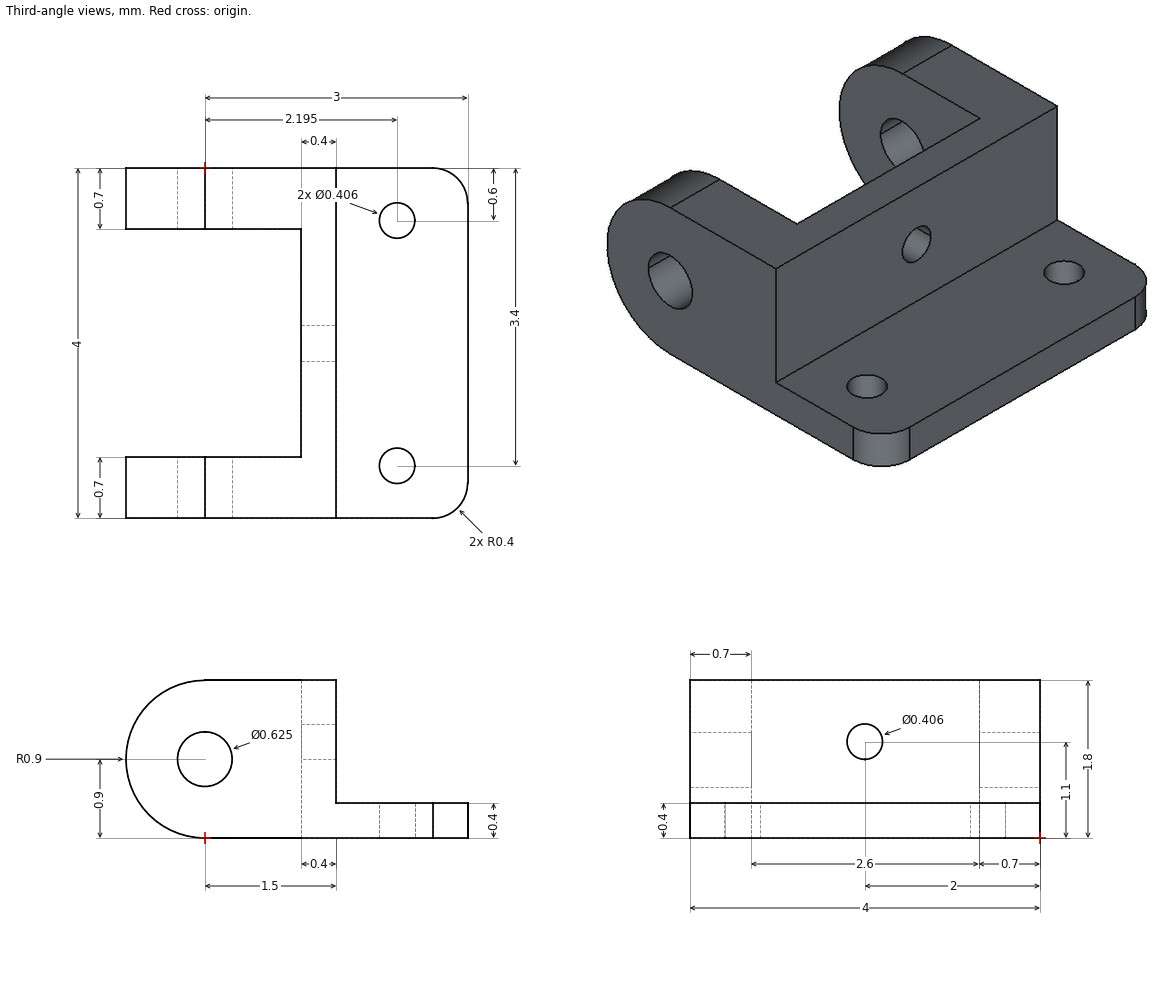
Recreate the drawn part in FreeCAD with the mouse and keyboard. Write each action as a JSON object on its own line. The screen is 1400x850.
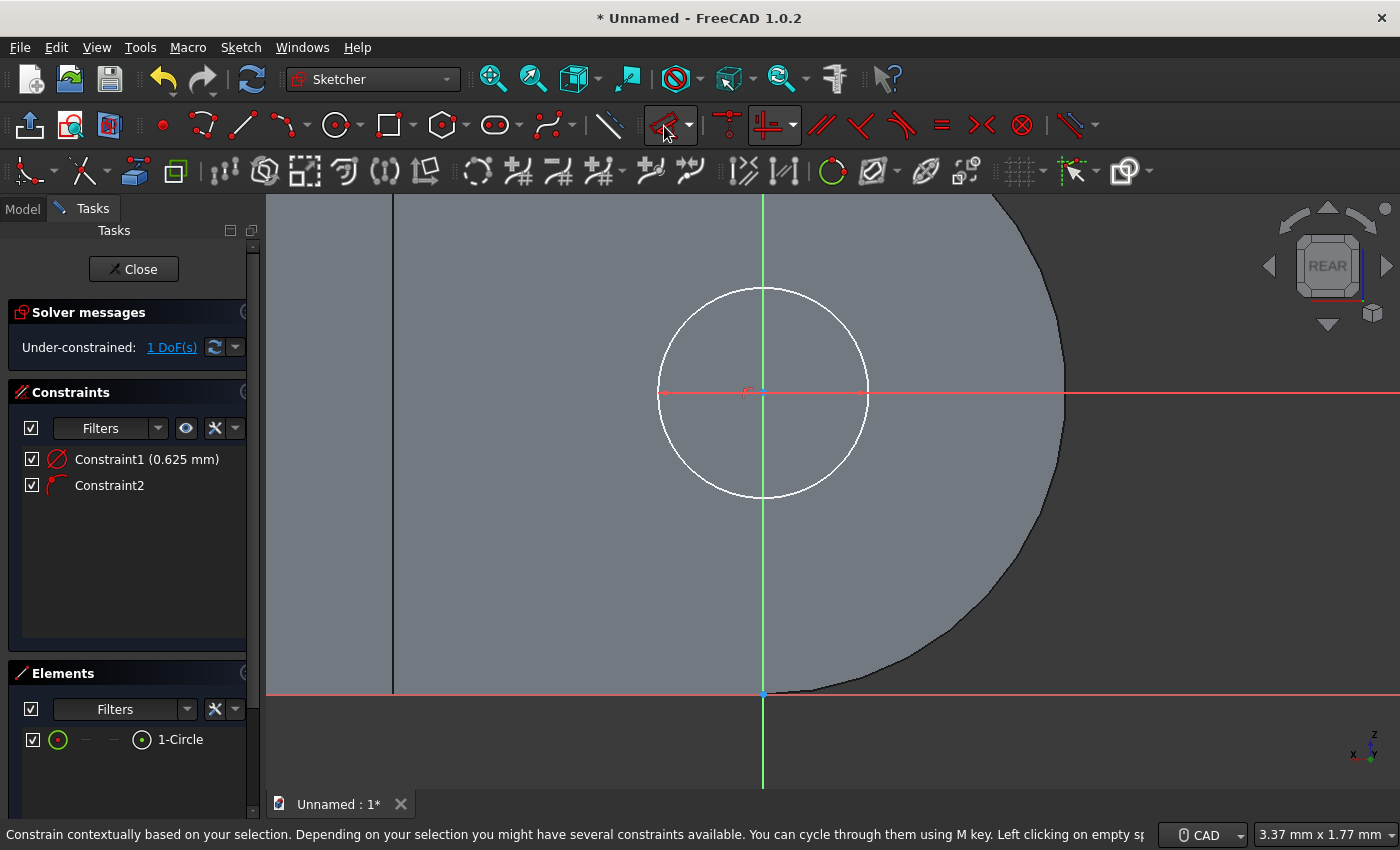
{"action": "left_click", "coordinate": [763, 393]}
{"action": "left_click", "coordinate": [797, 544]}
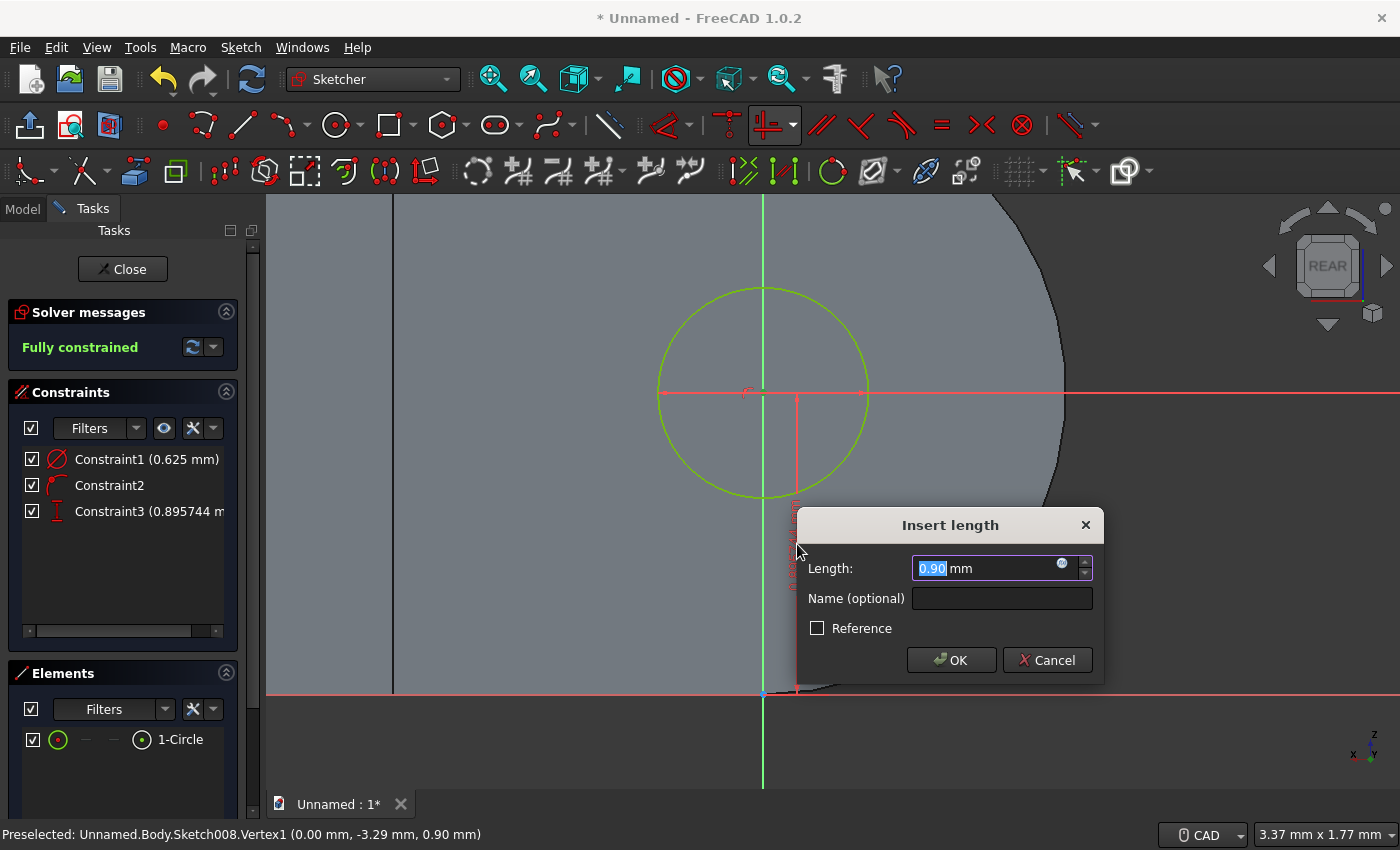
{"action": "type", "text": "0.9"}
{"action": "key", "text": "Return"}
{"action": "key", "text": "Escape"}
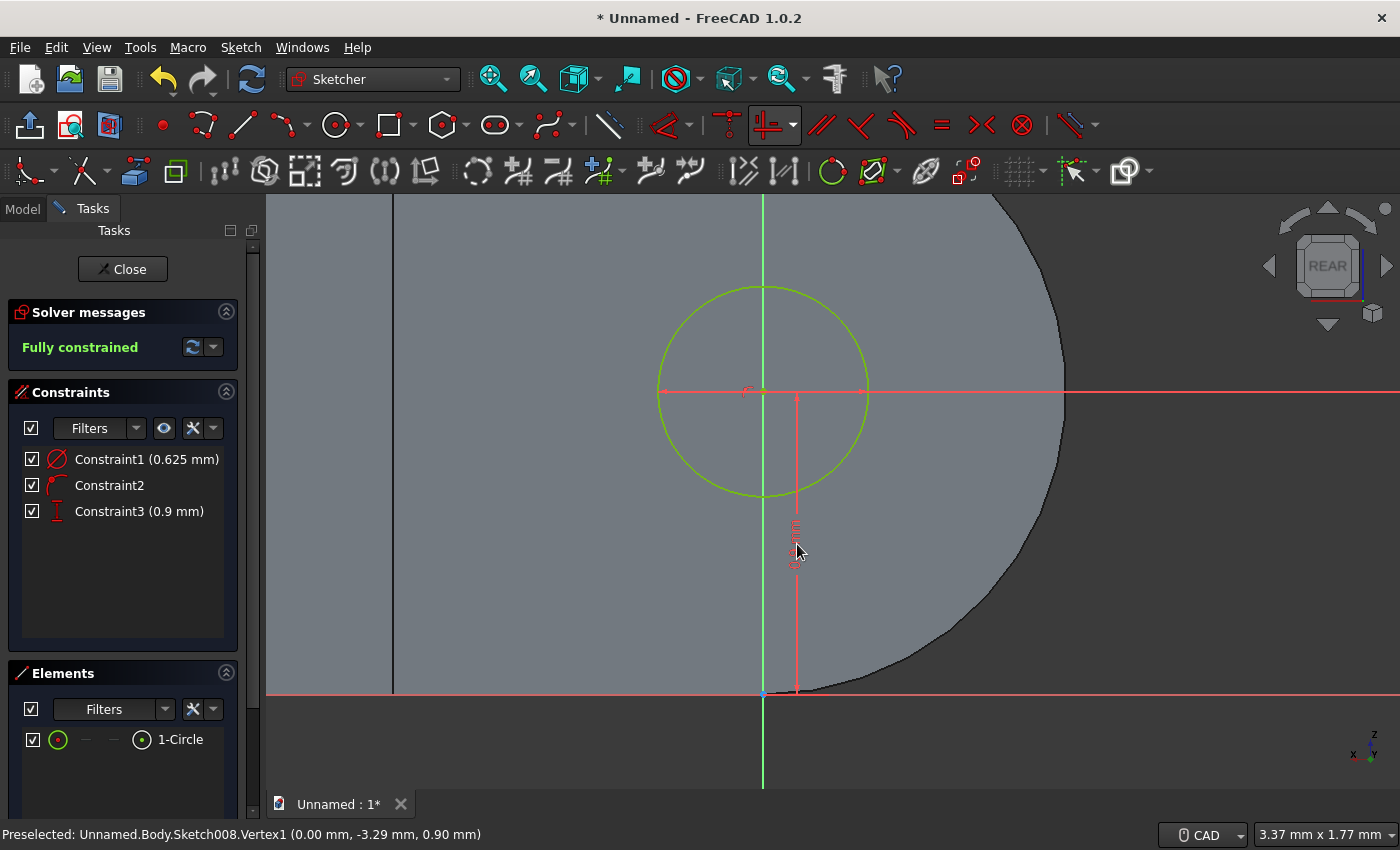
{"action": "left_click", "coordinate": [123, 269]}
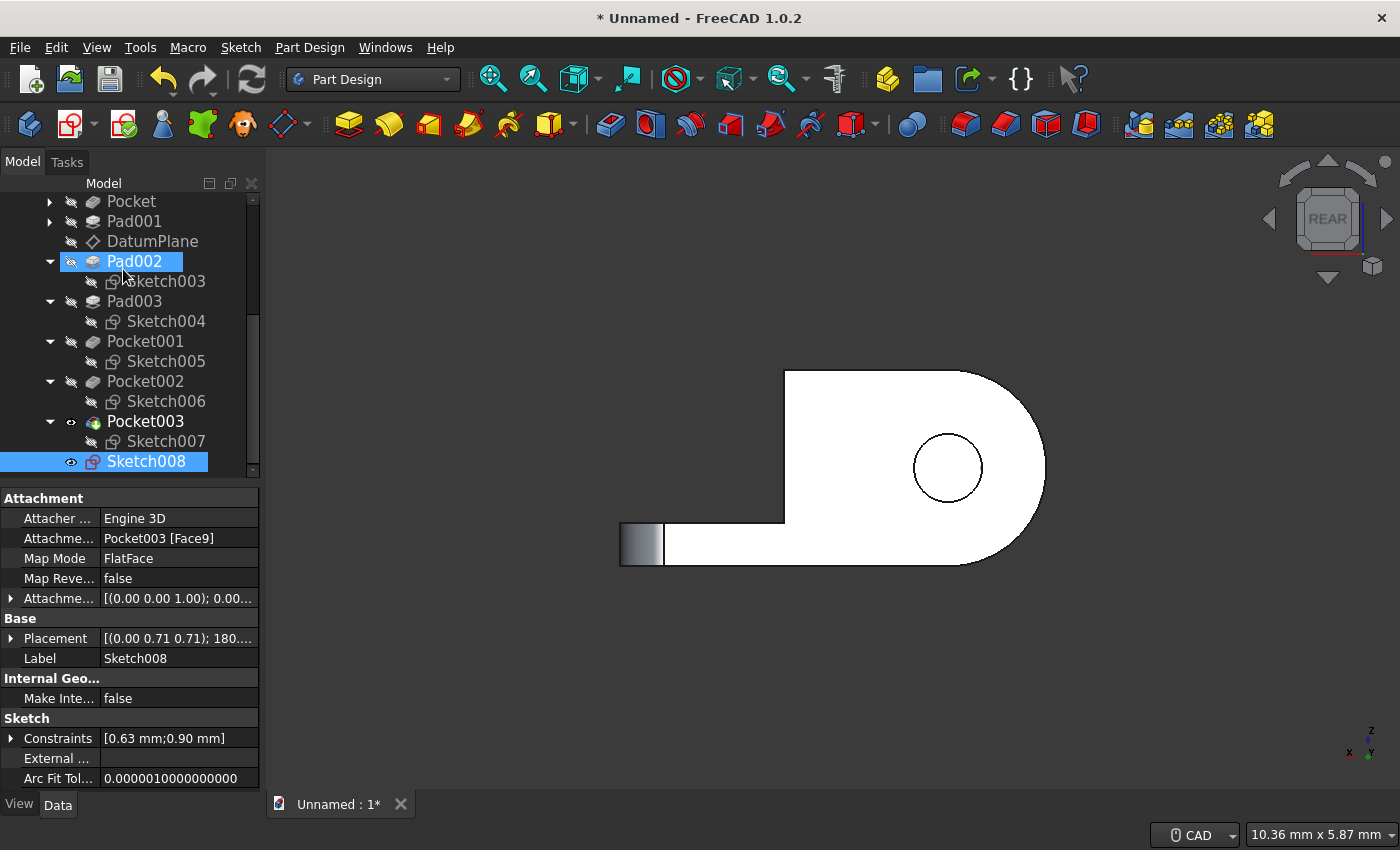
{"action": "left_click", "coordinate": [612, 124]}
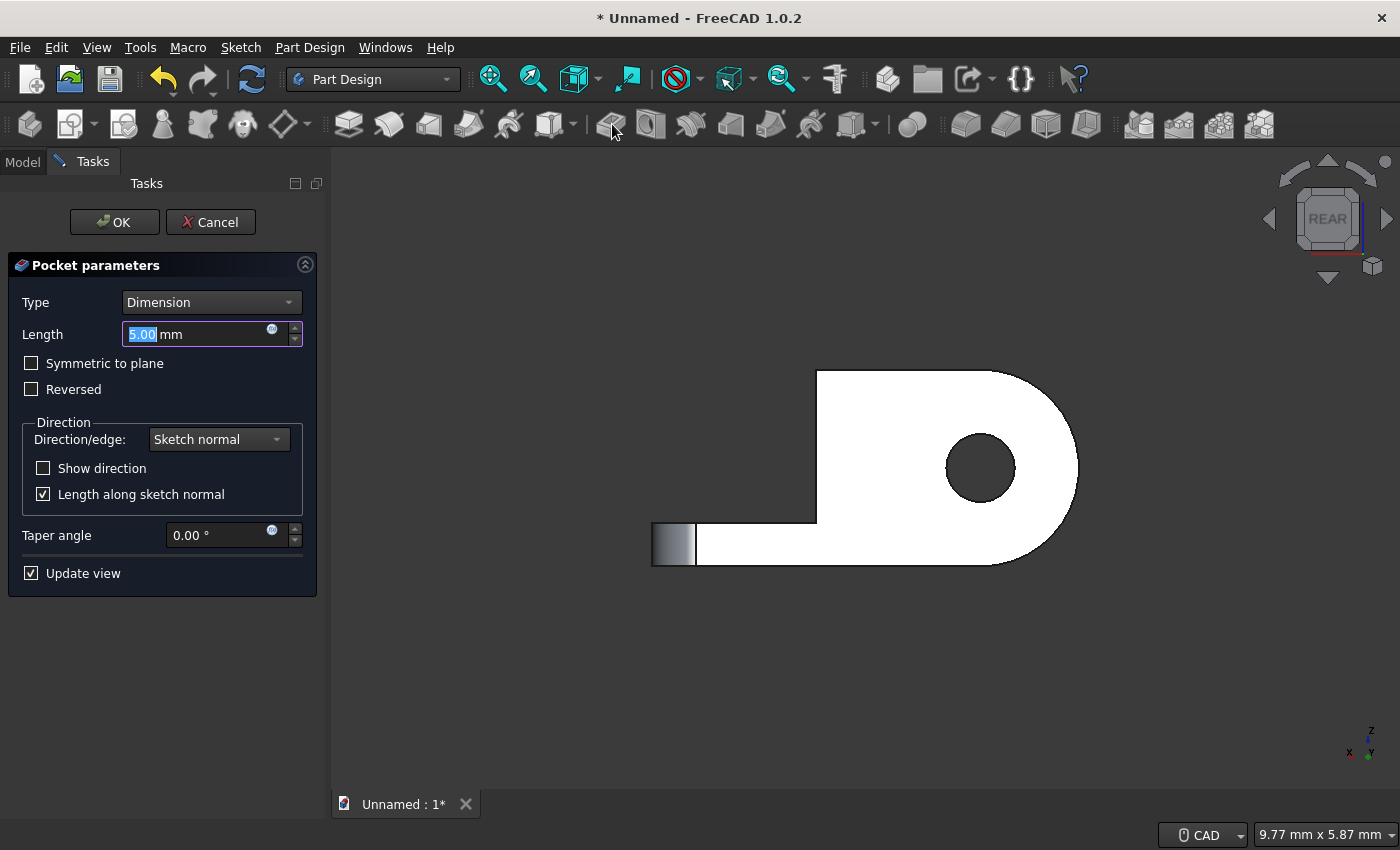
{"action": "type", "text": "0.7"}
{"action": "key", "text": "Tab"}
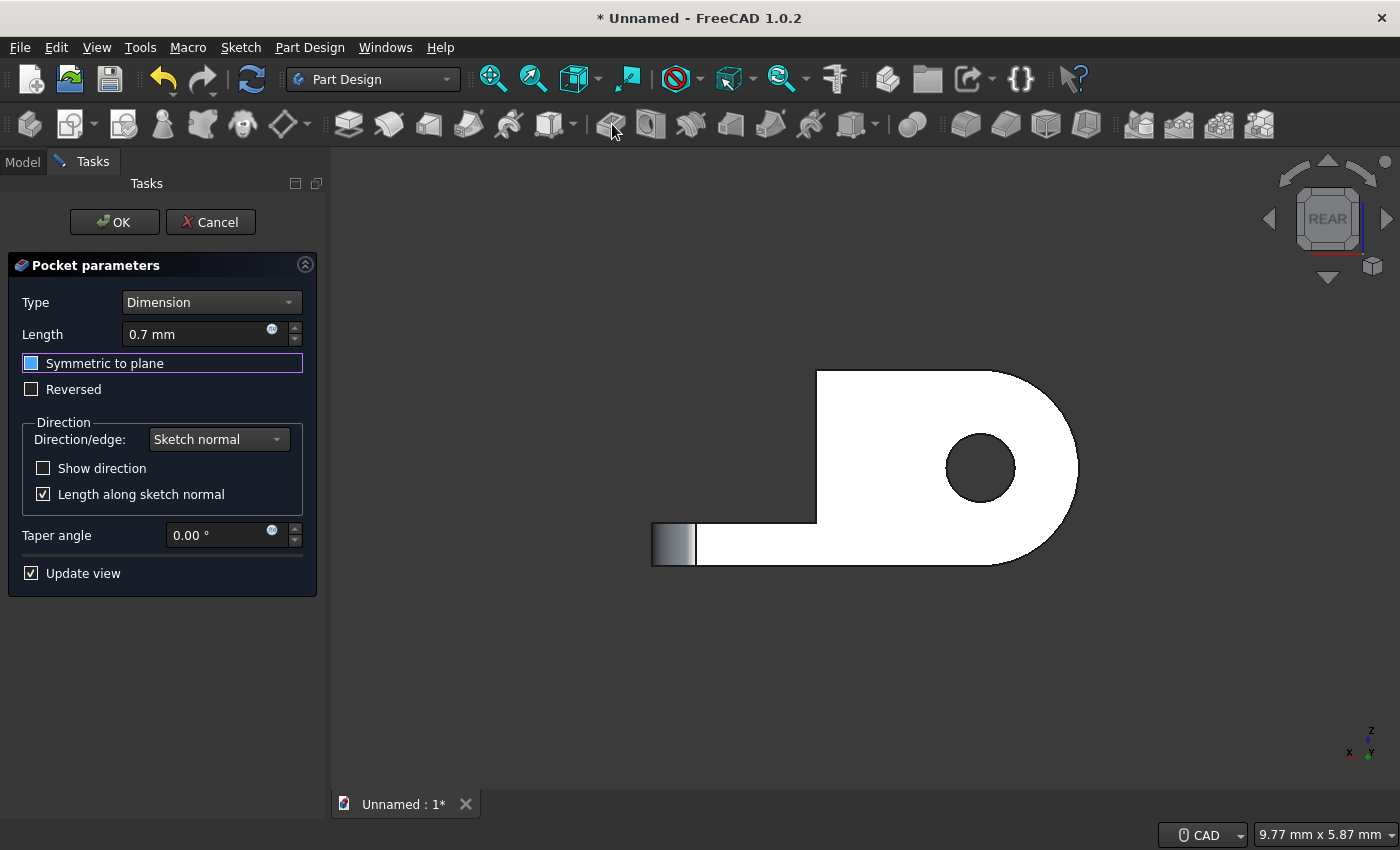
{"action": "left_click", "coordinate": [115, 222]}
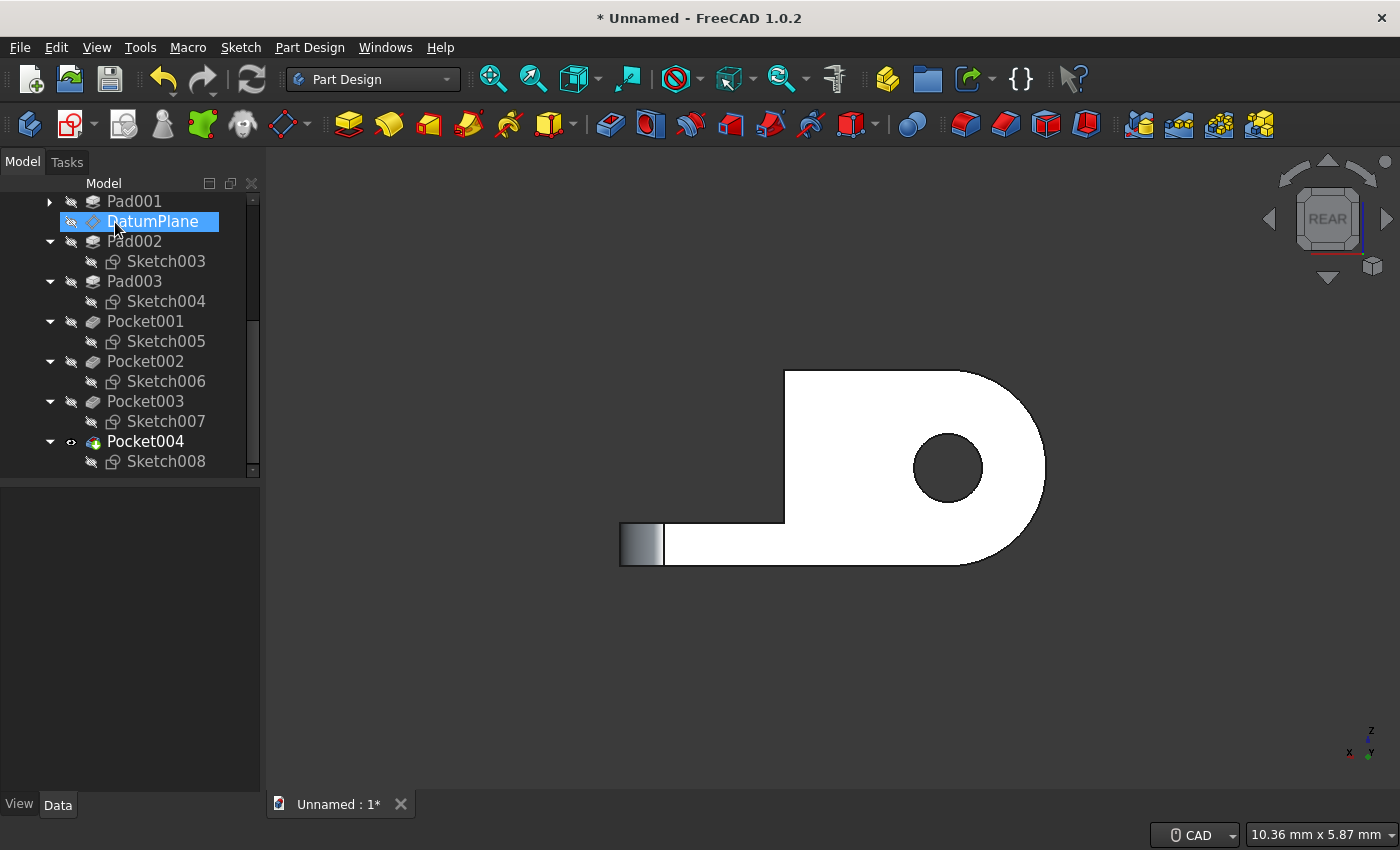
{"action": "key", "text": "0"}